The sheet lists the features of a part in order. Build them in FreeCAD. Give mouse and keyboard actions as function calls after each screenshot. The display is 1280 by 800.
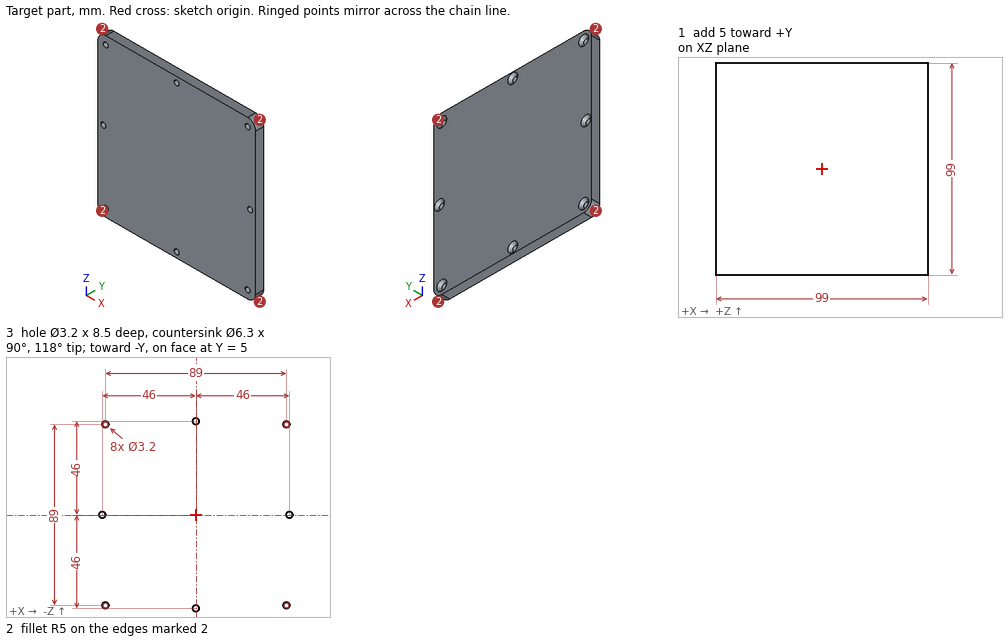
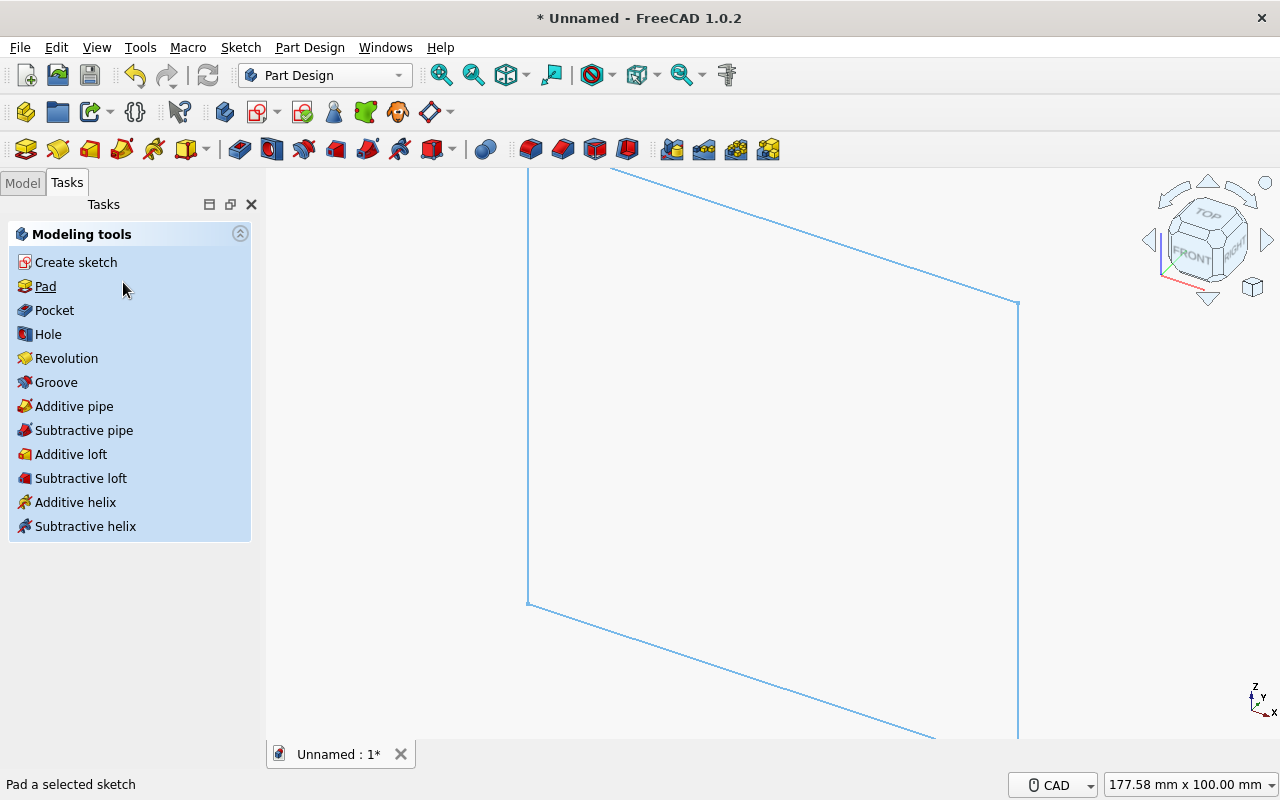
click(26, 150)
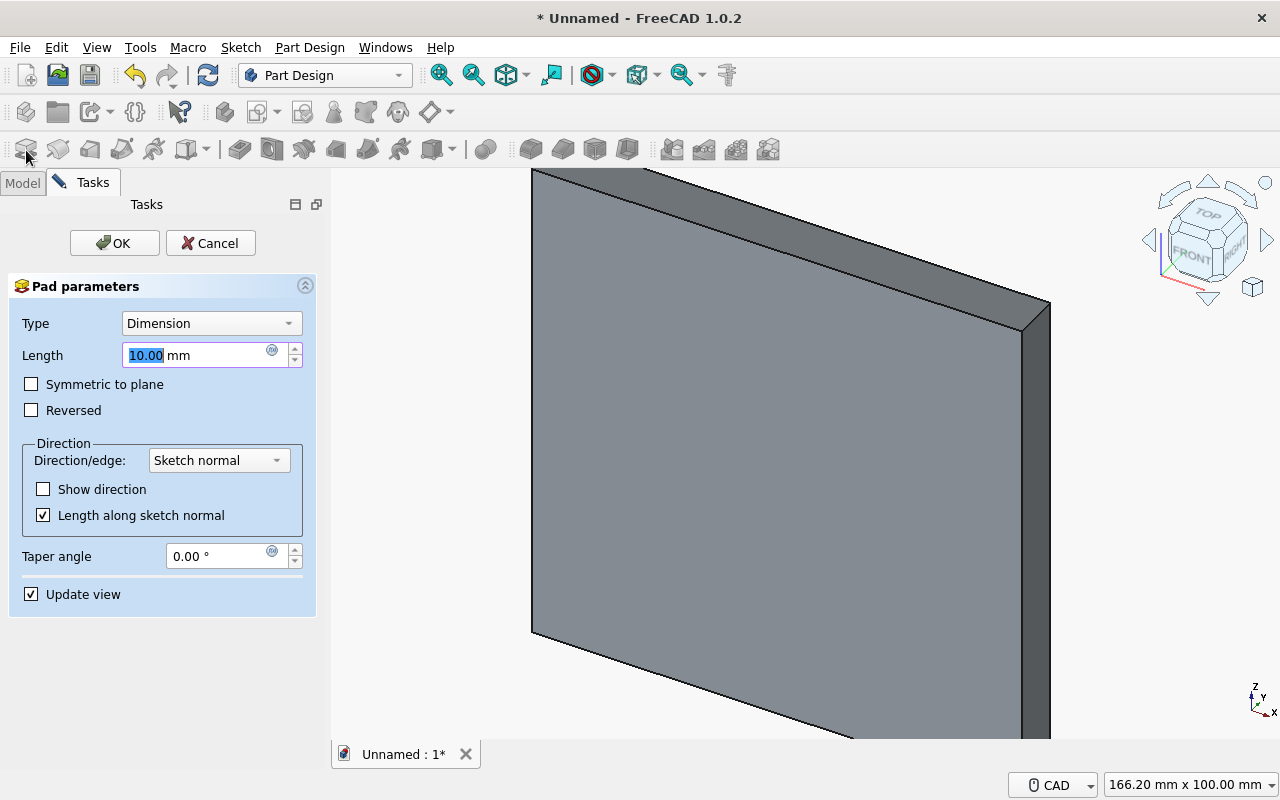
text(5)
key(Tab)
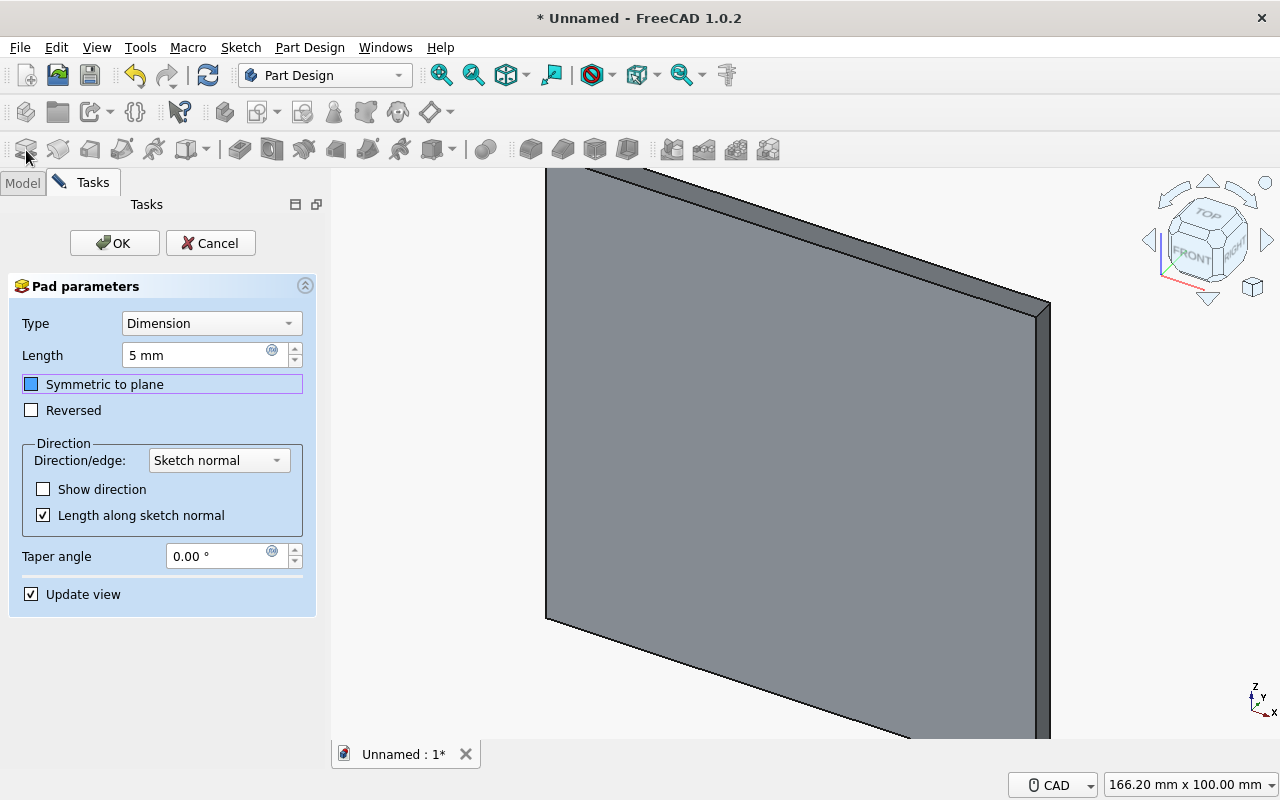
click(30, 410)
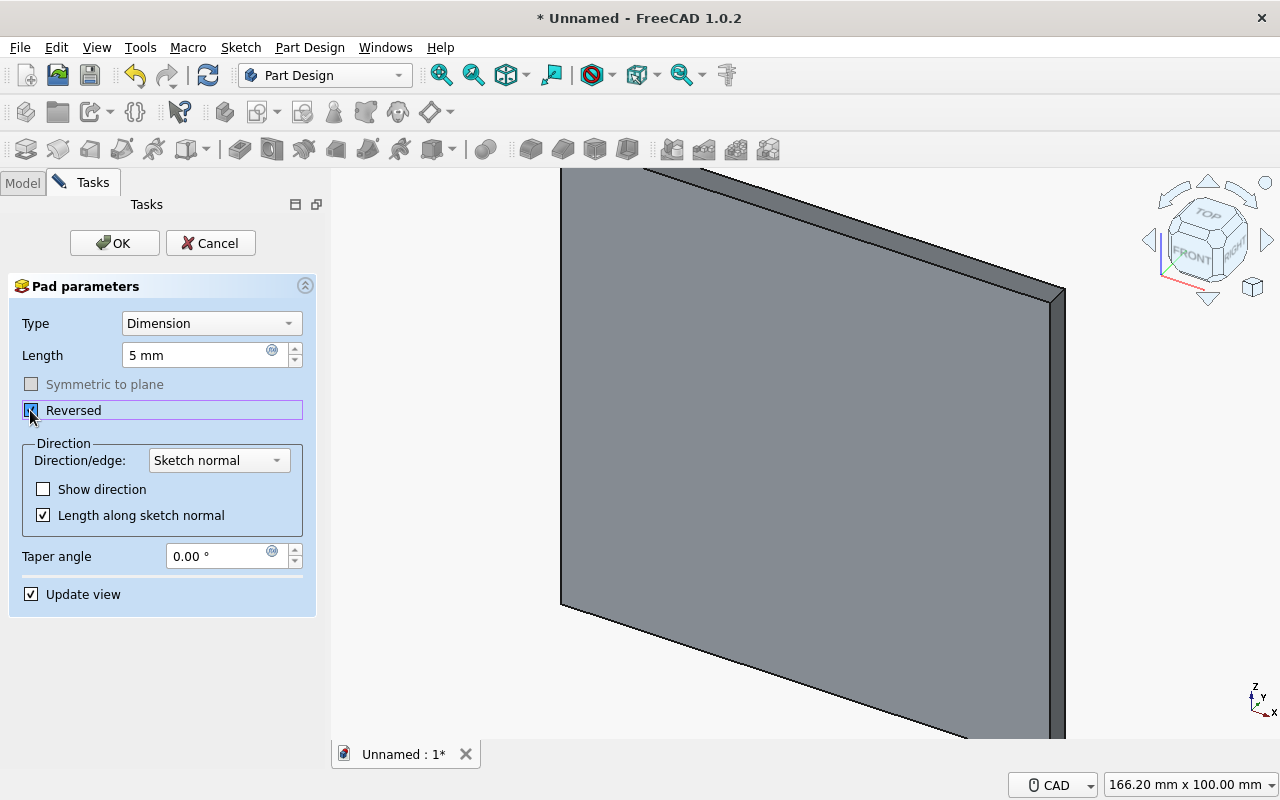
click(115, 243)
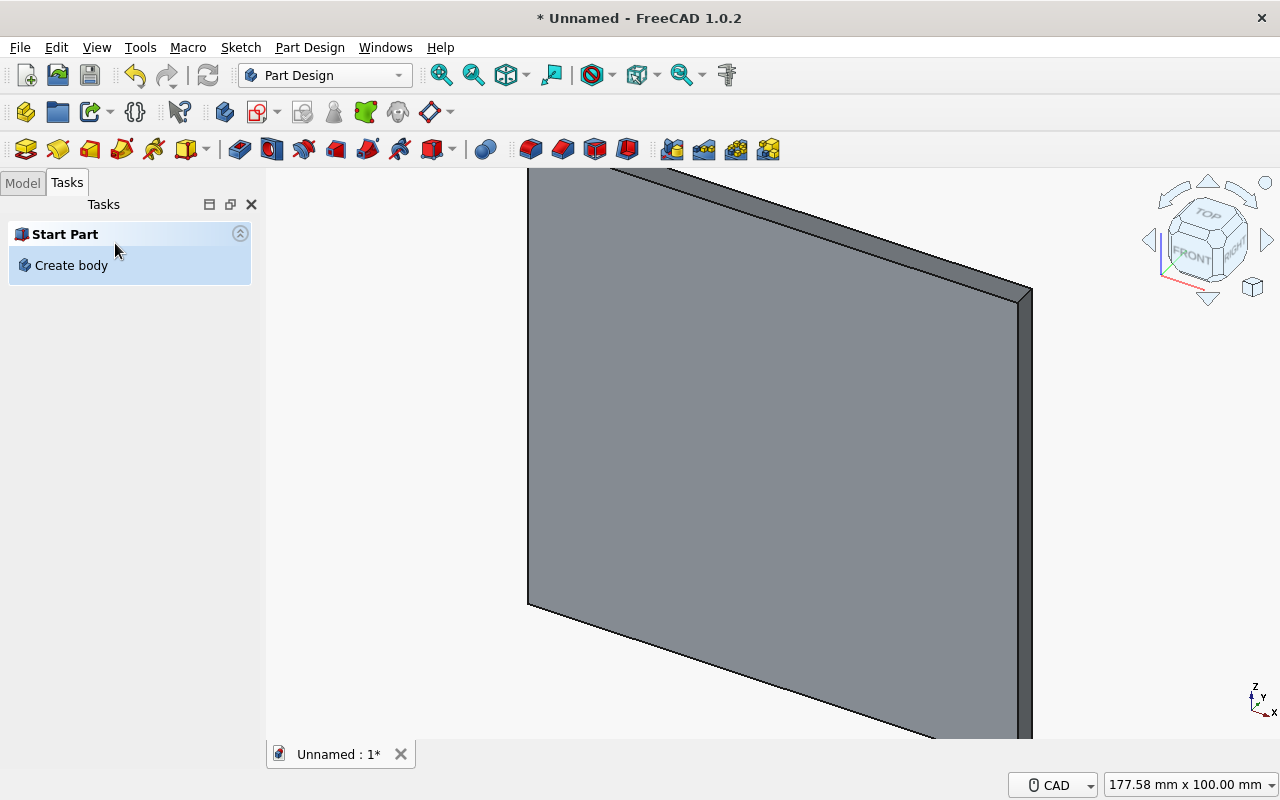
click(442, 76)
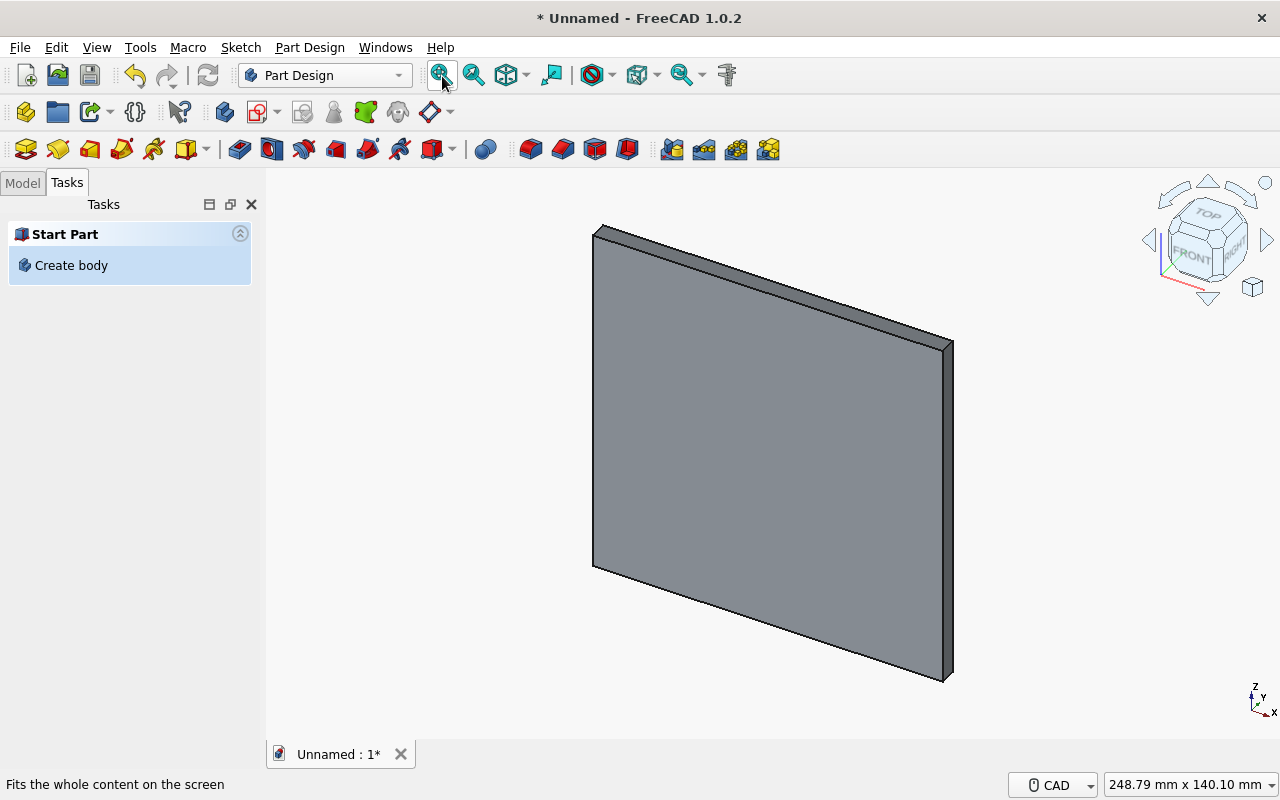
click(948, 345)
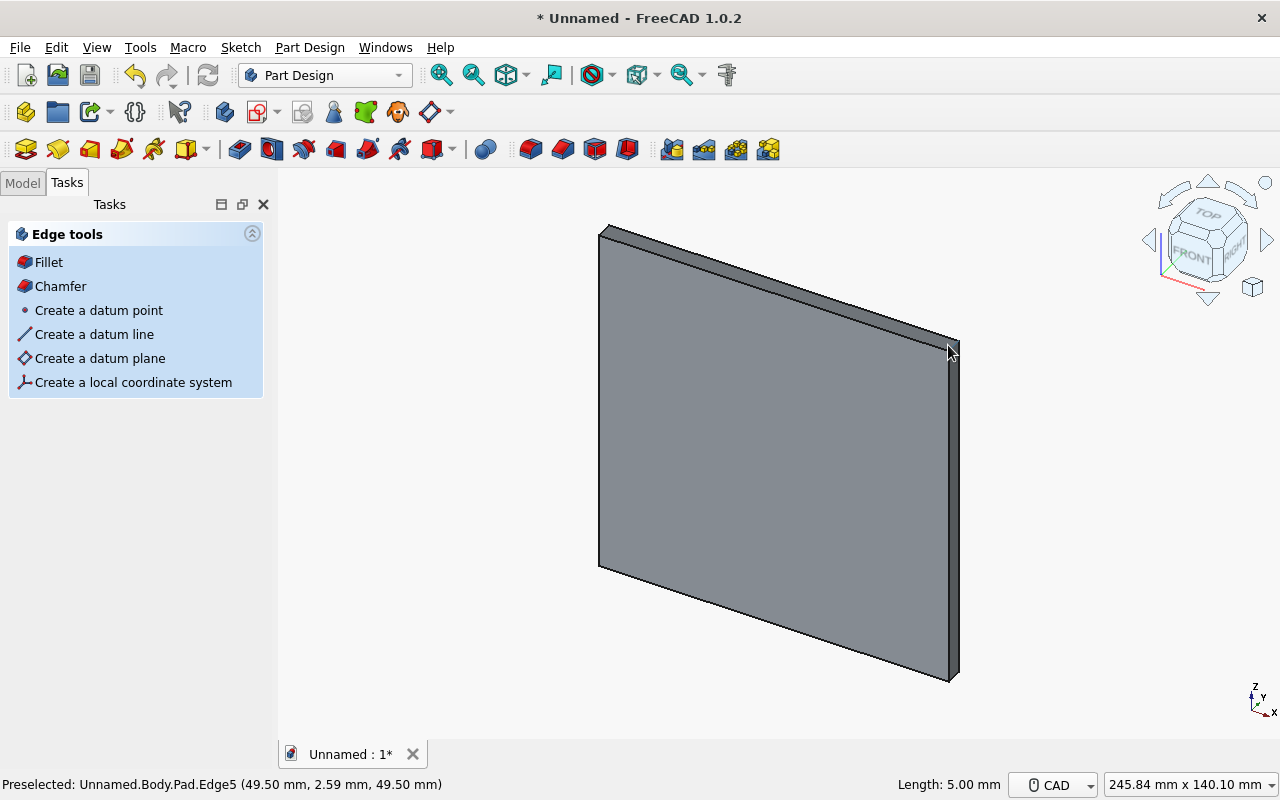
scroll(604, 229, up, 4)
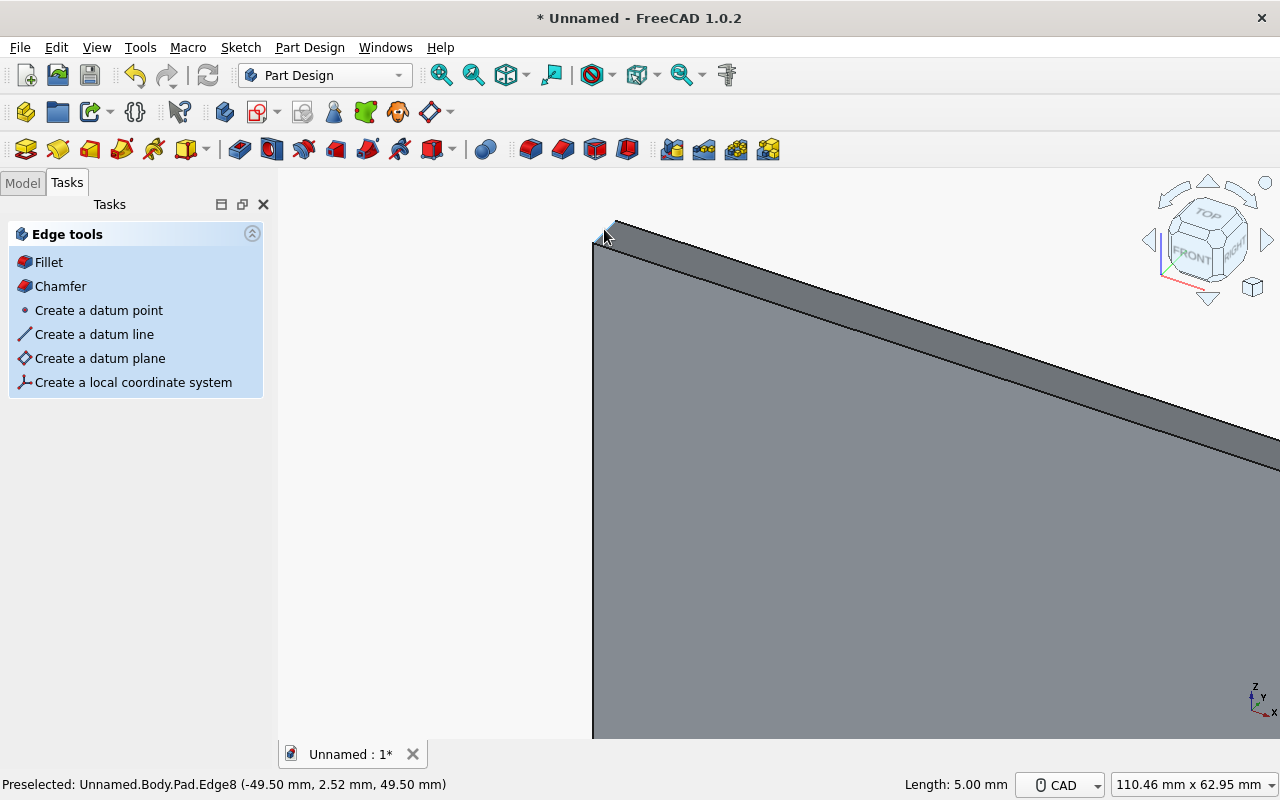
key(v)
key(f)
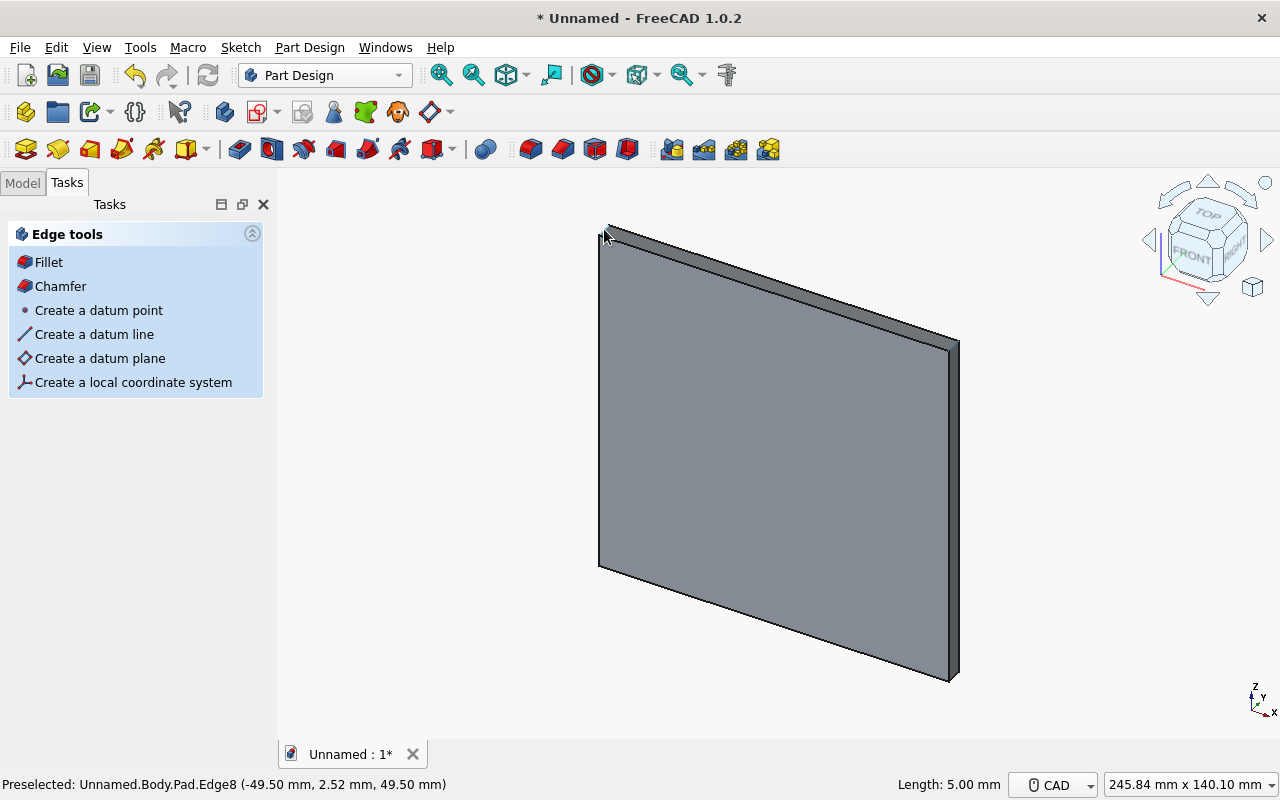
key(0)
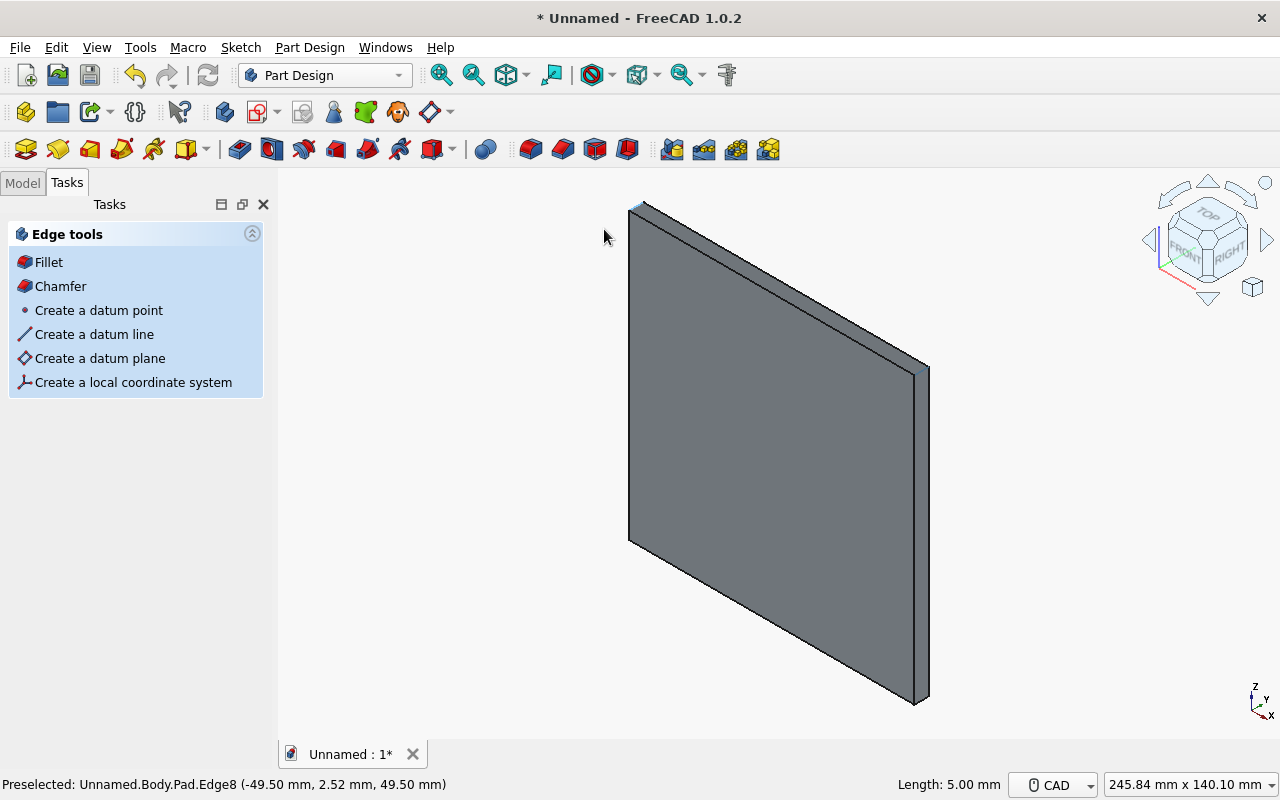
scroll(636, 205, up, 4)